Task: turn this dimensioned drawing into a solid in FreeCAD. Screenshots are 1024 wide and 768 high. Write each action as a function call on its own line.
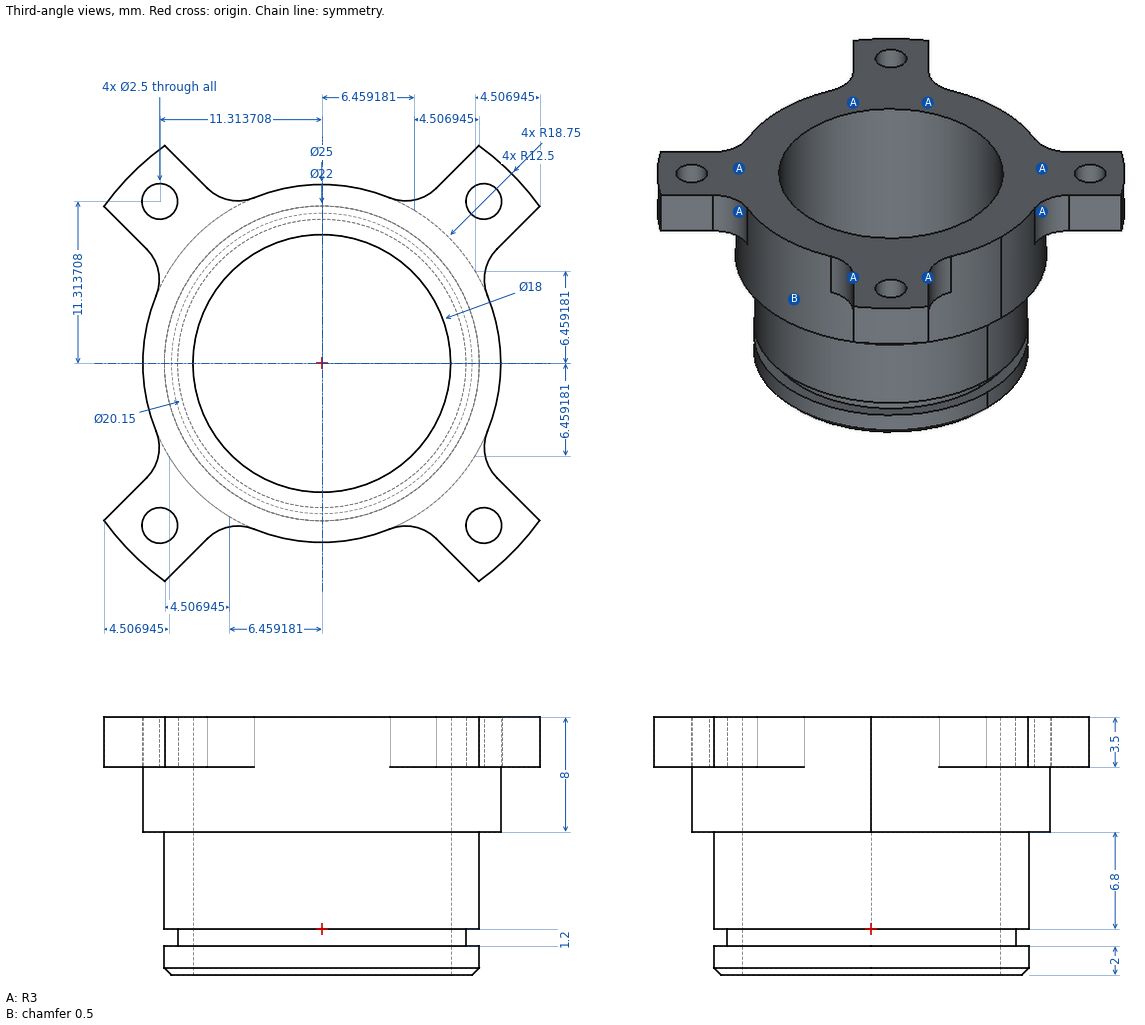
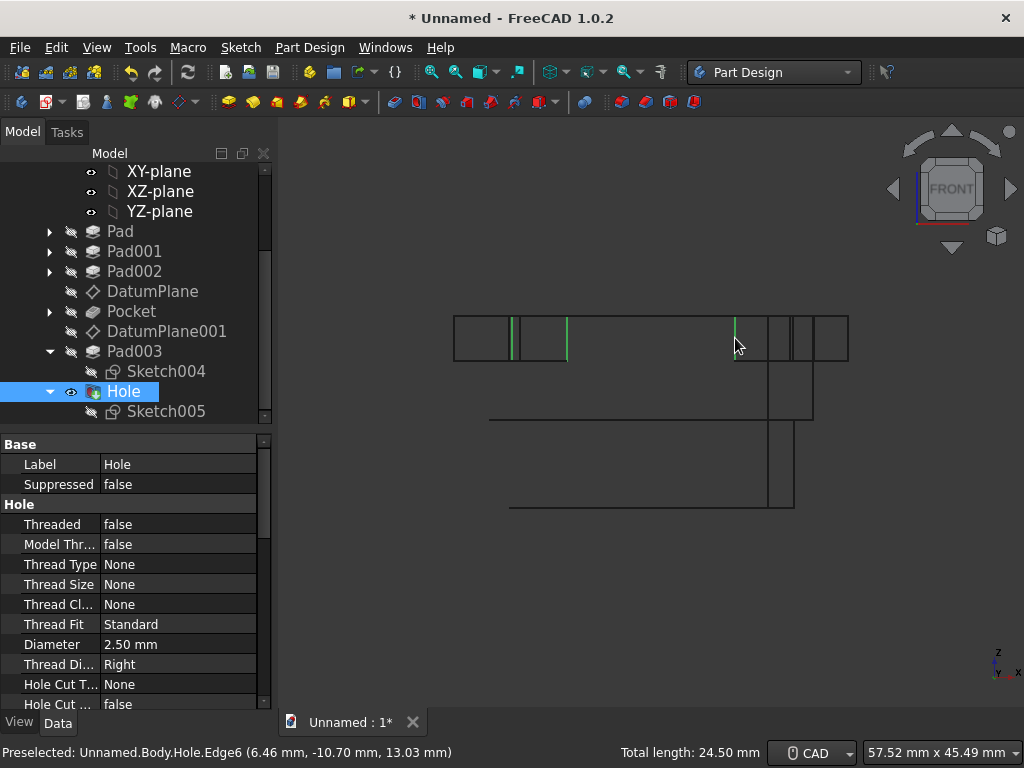
key(3)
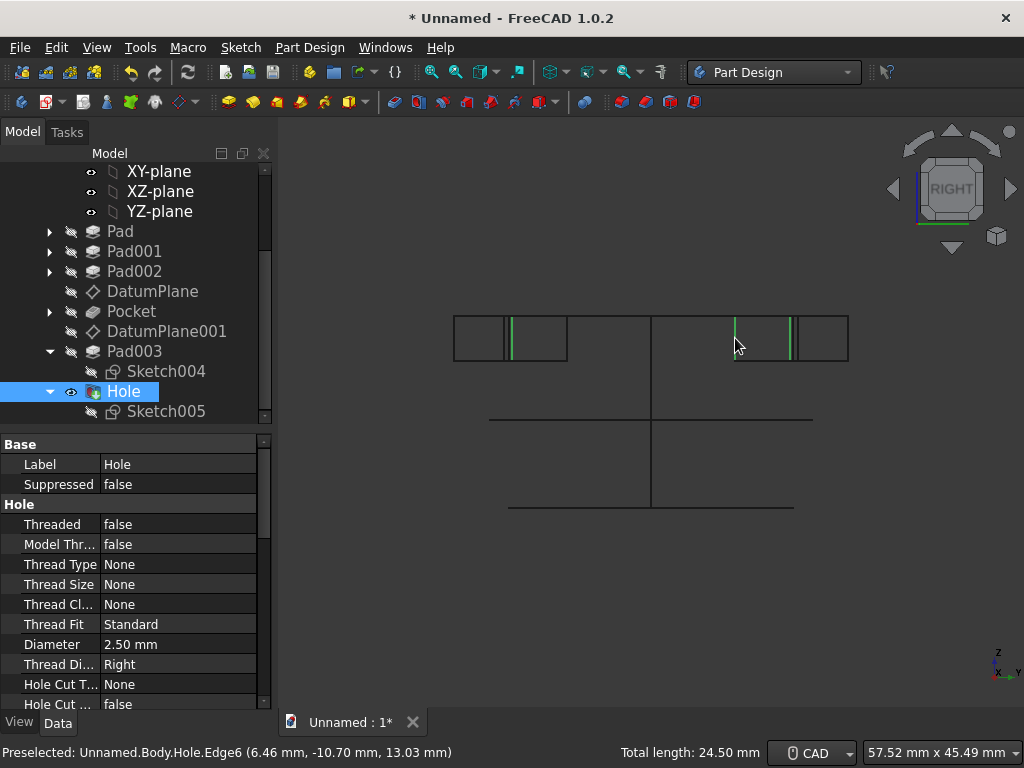
click(567, 338, ctrl)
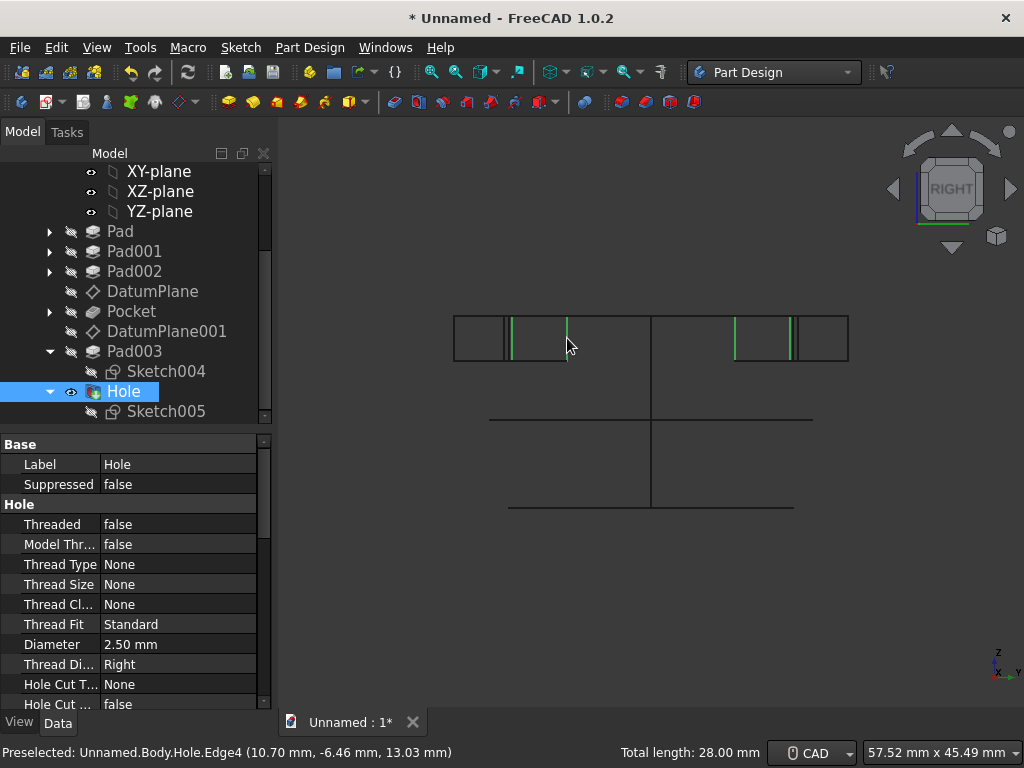
key(v)
key(1)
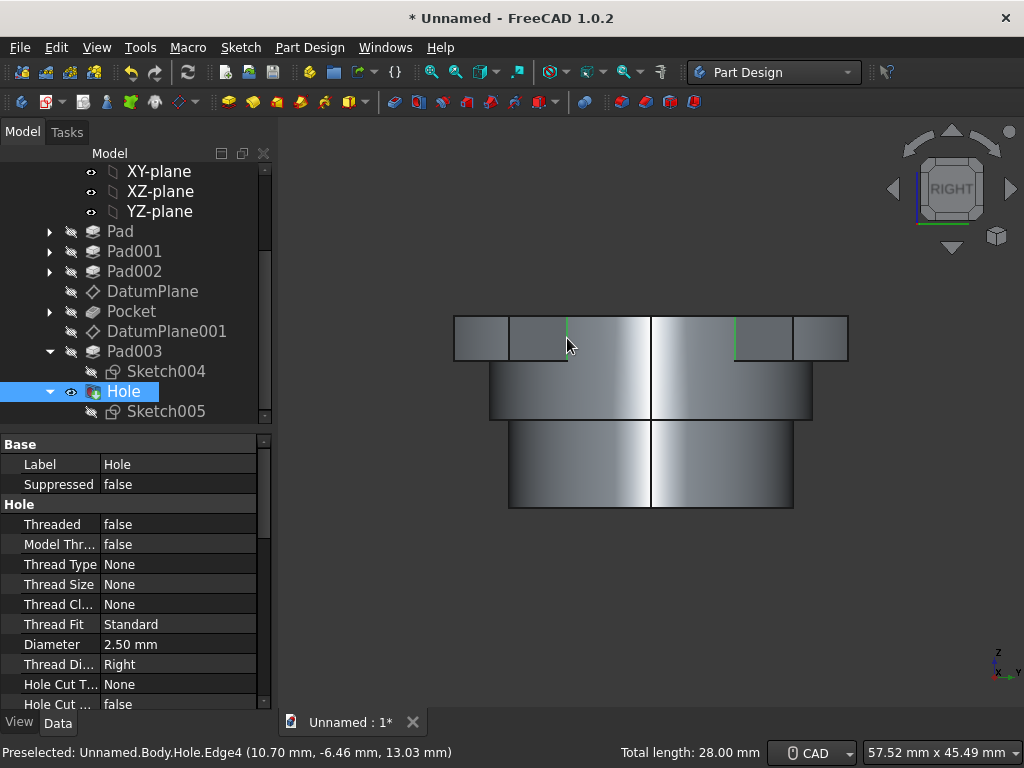
click(622, 102)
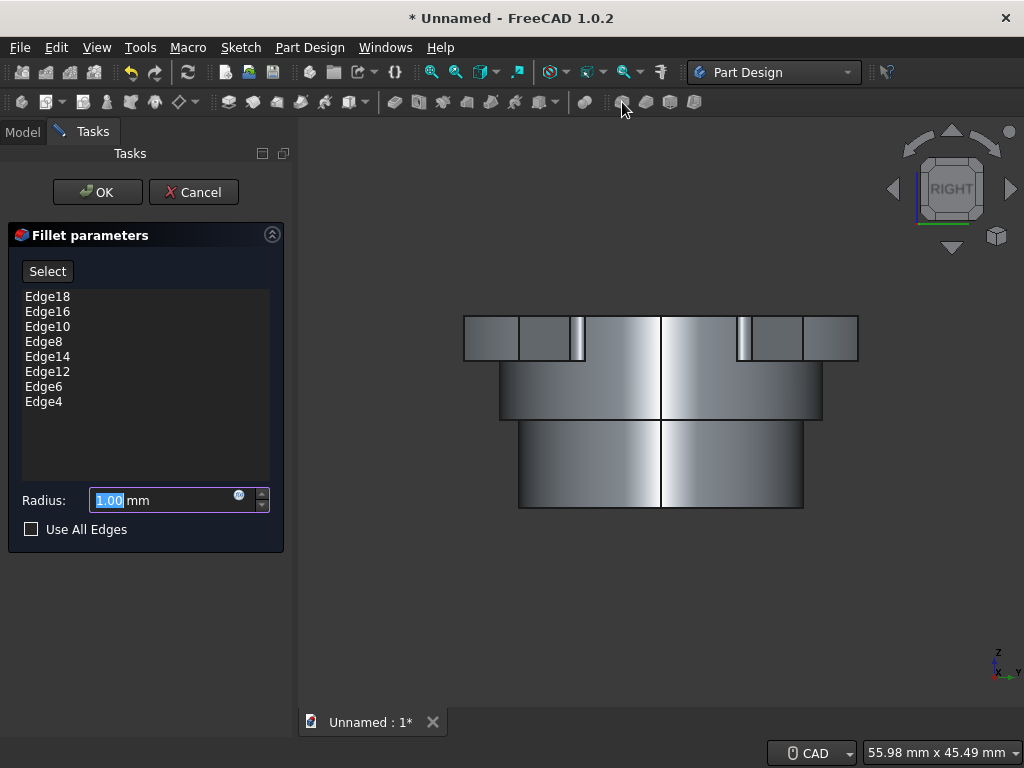
text(3)
key(Tab)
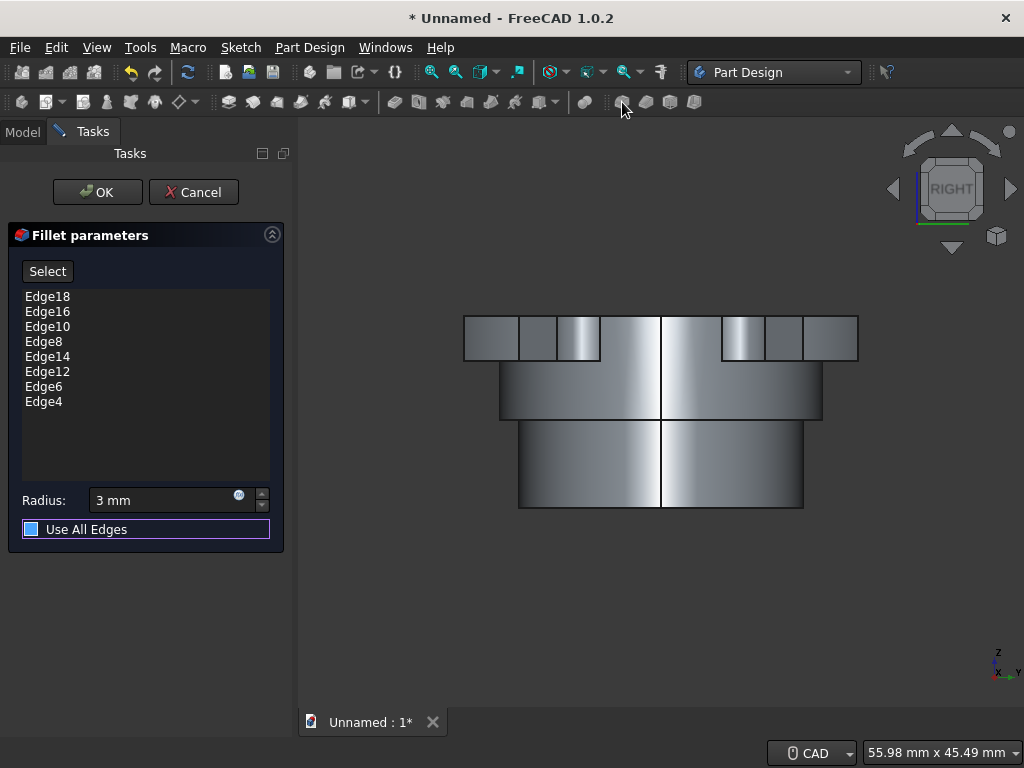
click(98, 192)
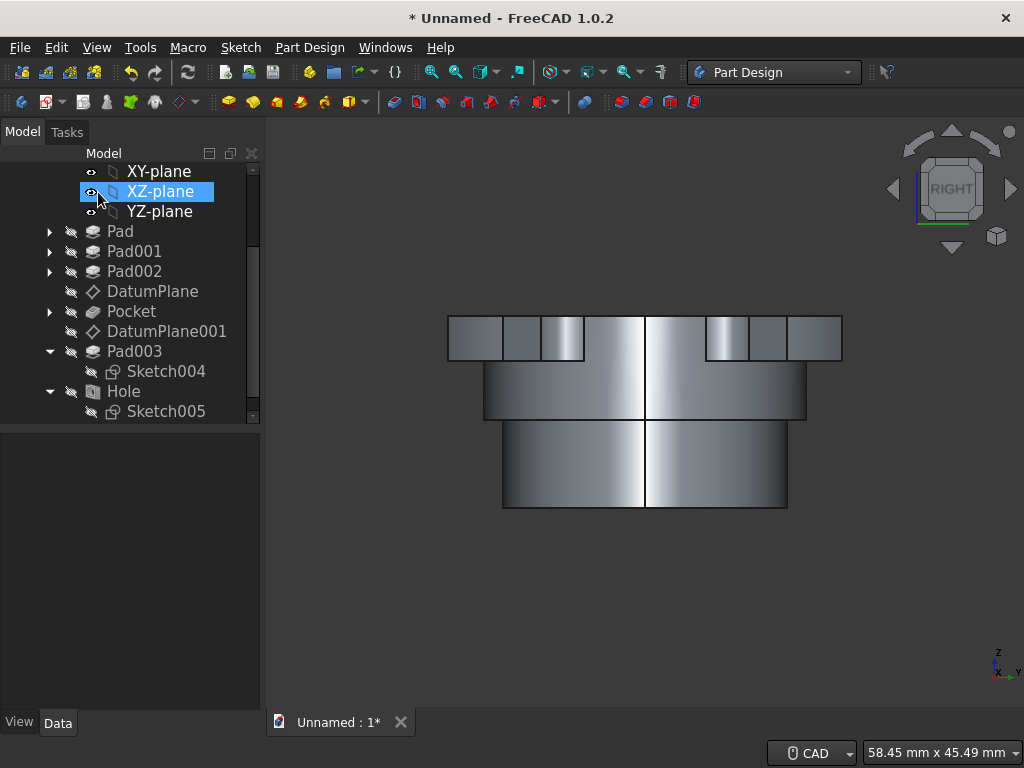
scroll(160, 287, down, 3)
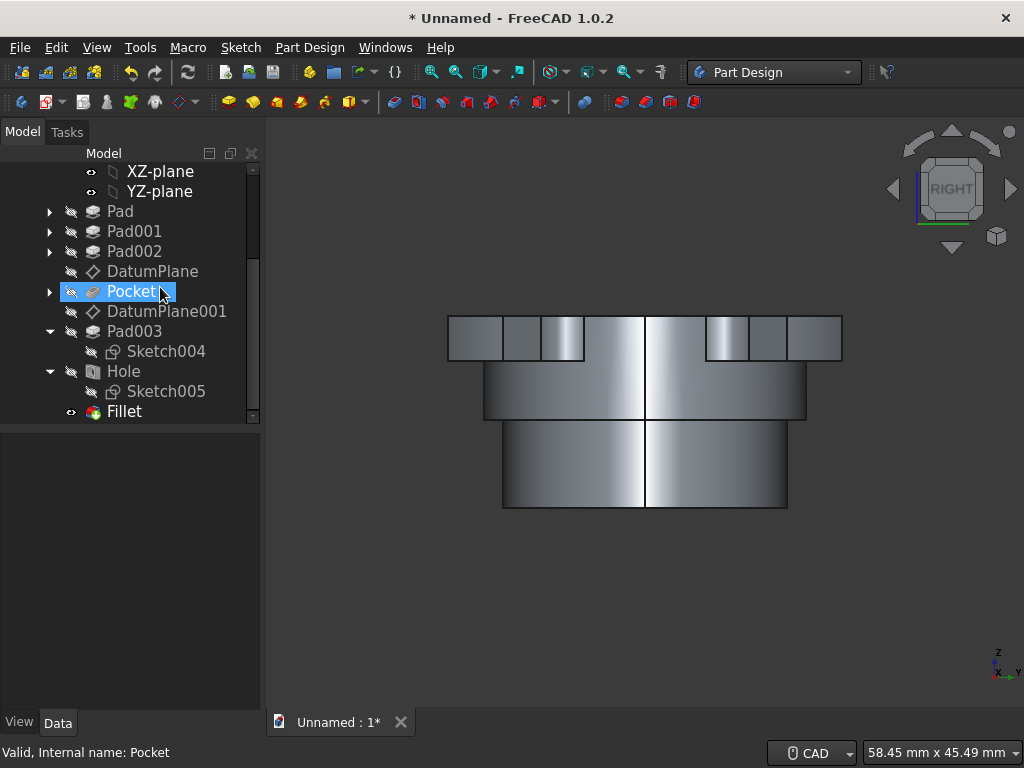
scroll(160, 287, up, 15)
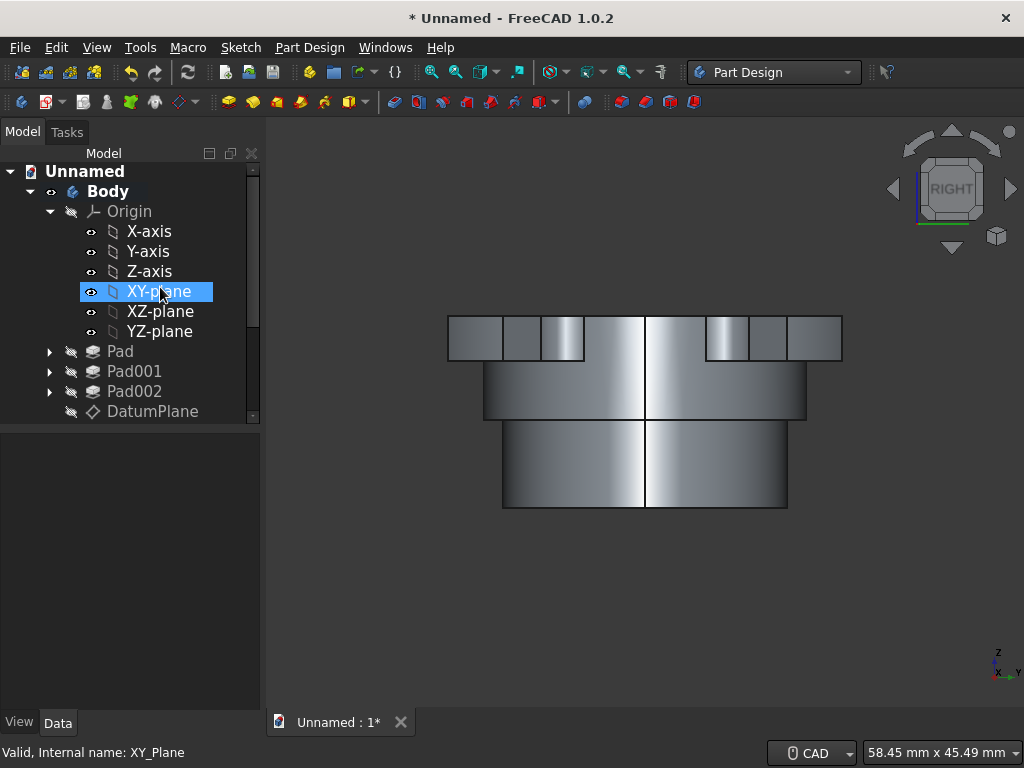
click(136, 292)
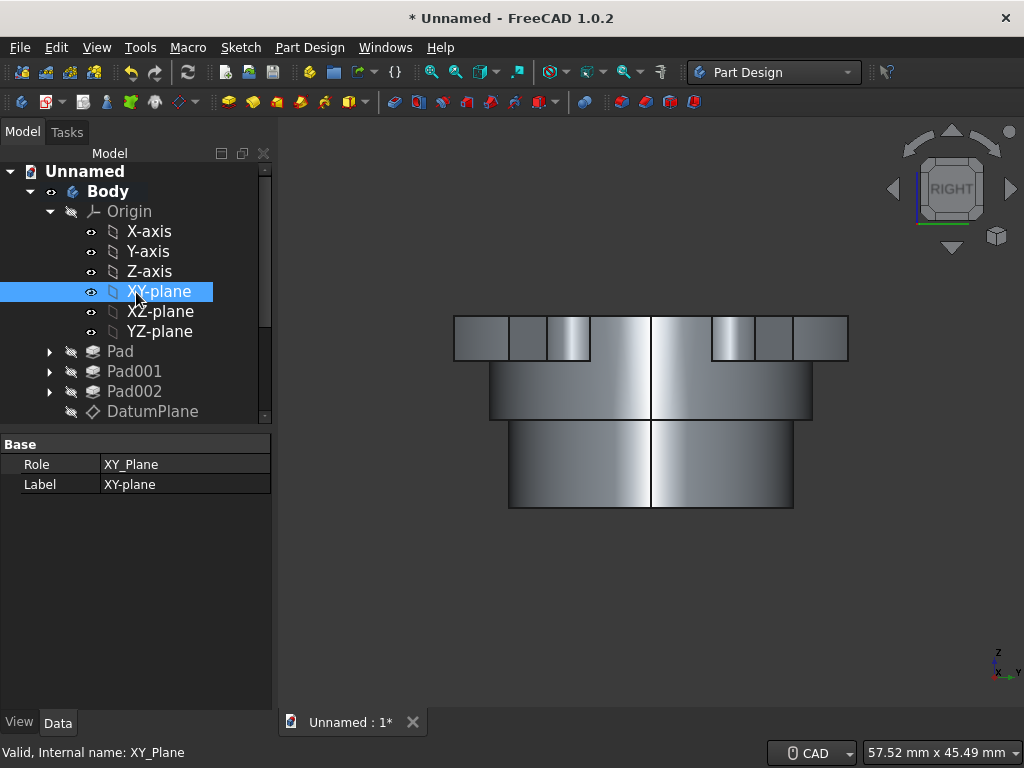
click(180, 102)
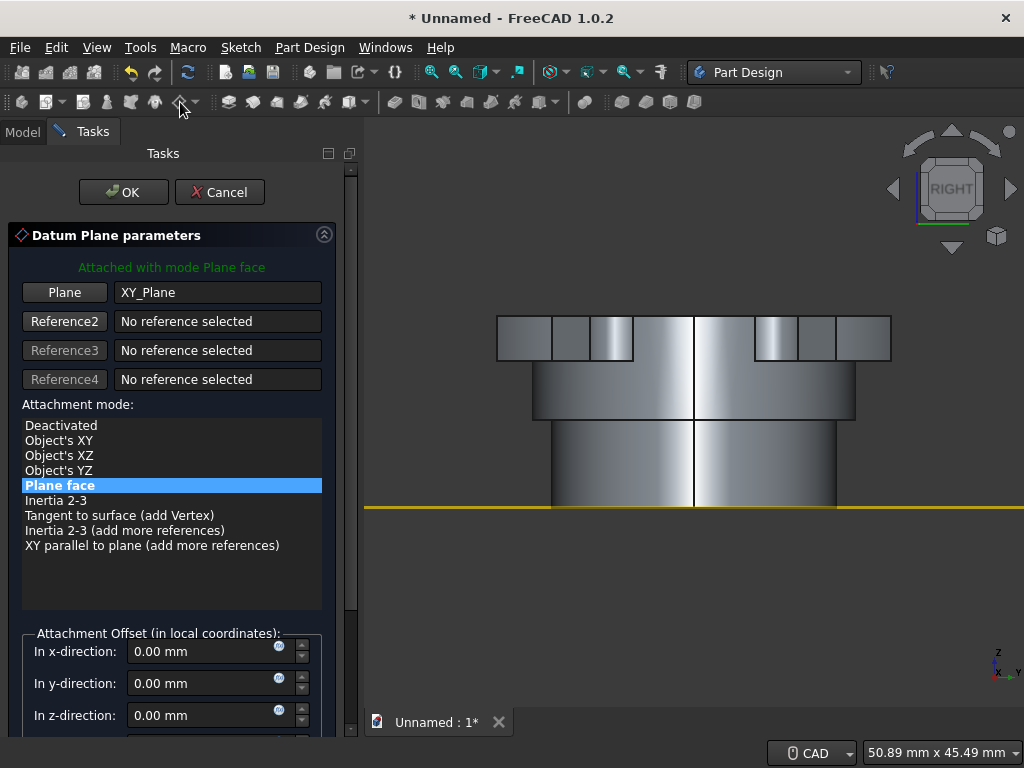
triple_click(210, 715)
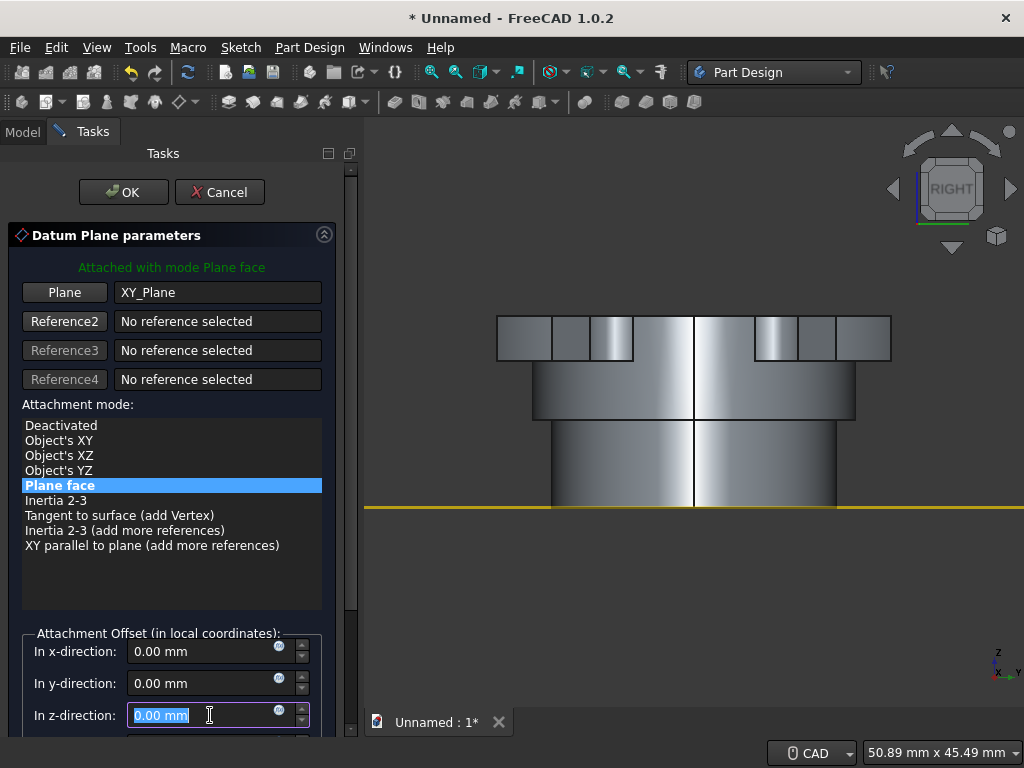
text(-1.2)
key(Tab)